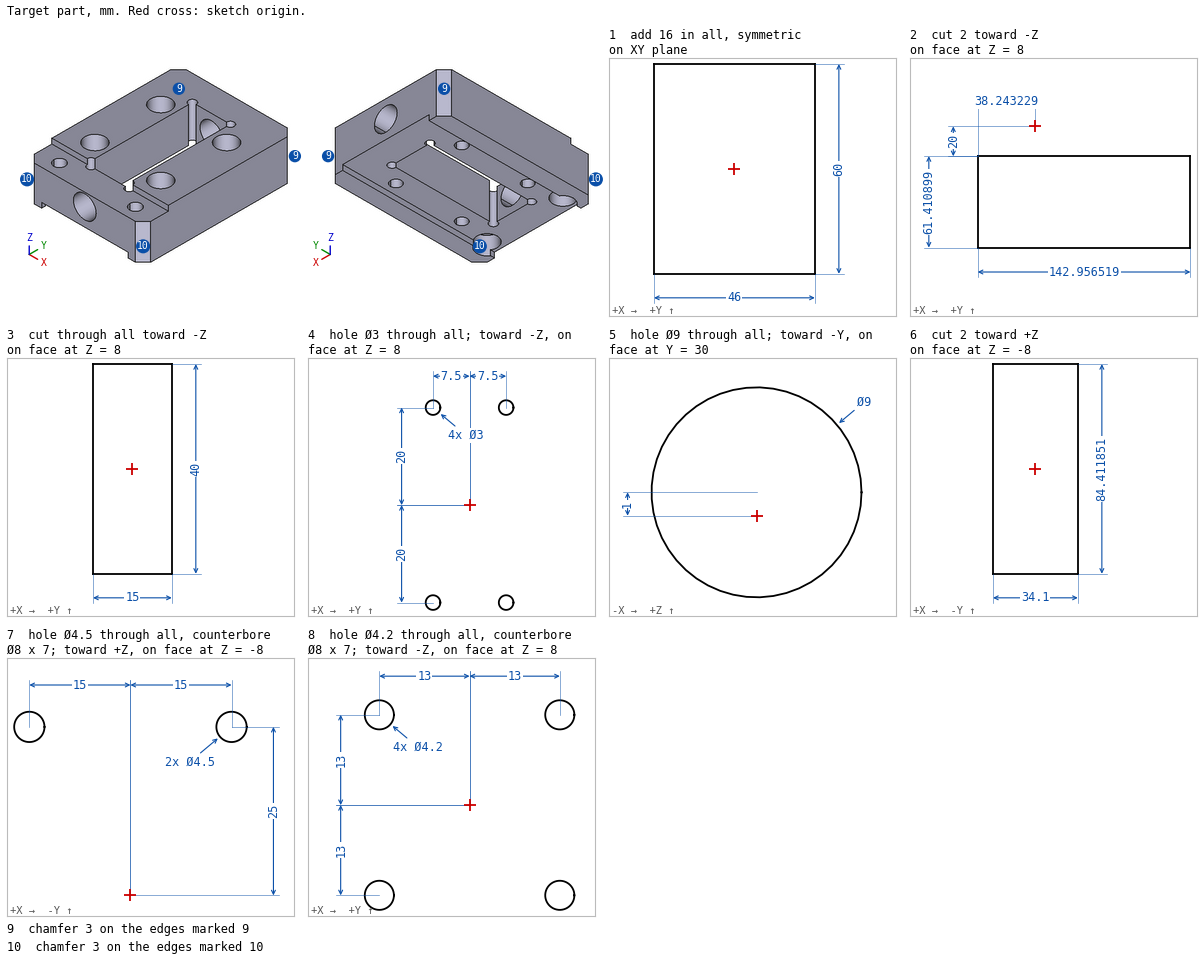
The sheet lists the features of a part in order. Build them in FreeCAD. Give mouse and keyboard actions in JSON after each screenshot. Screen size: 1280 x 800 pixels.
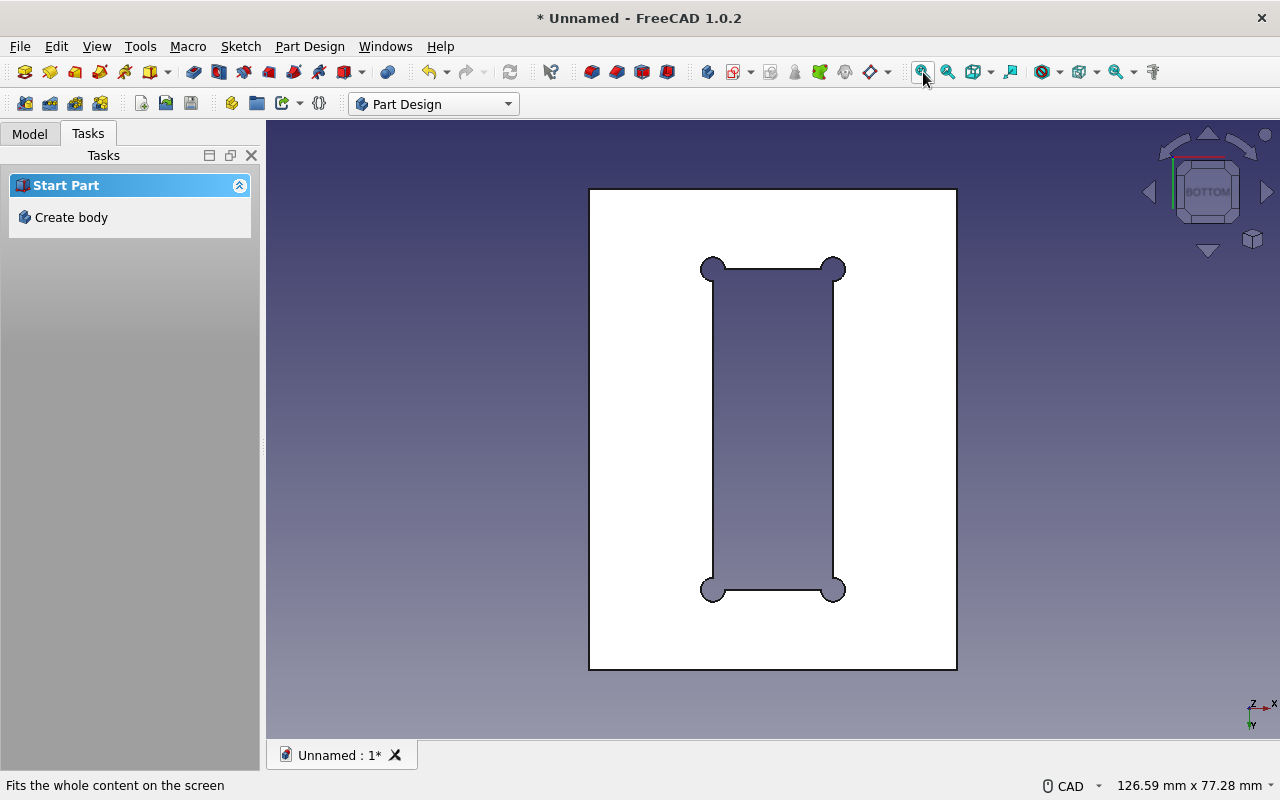
{"action": "left_click", "coordinate": [878, 497]}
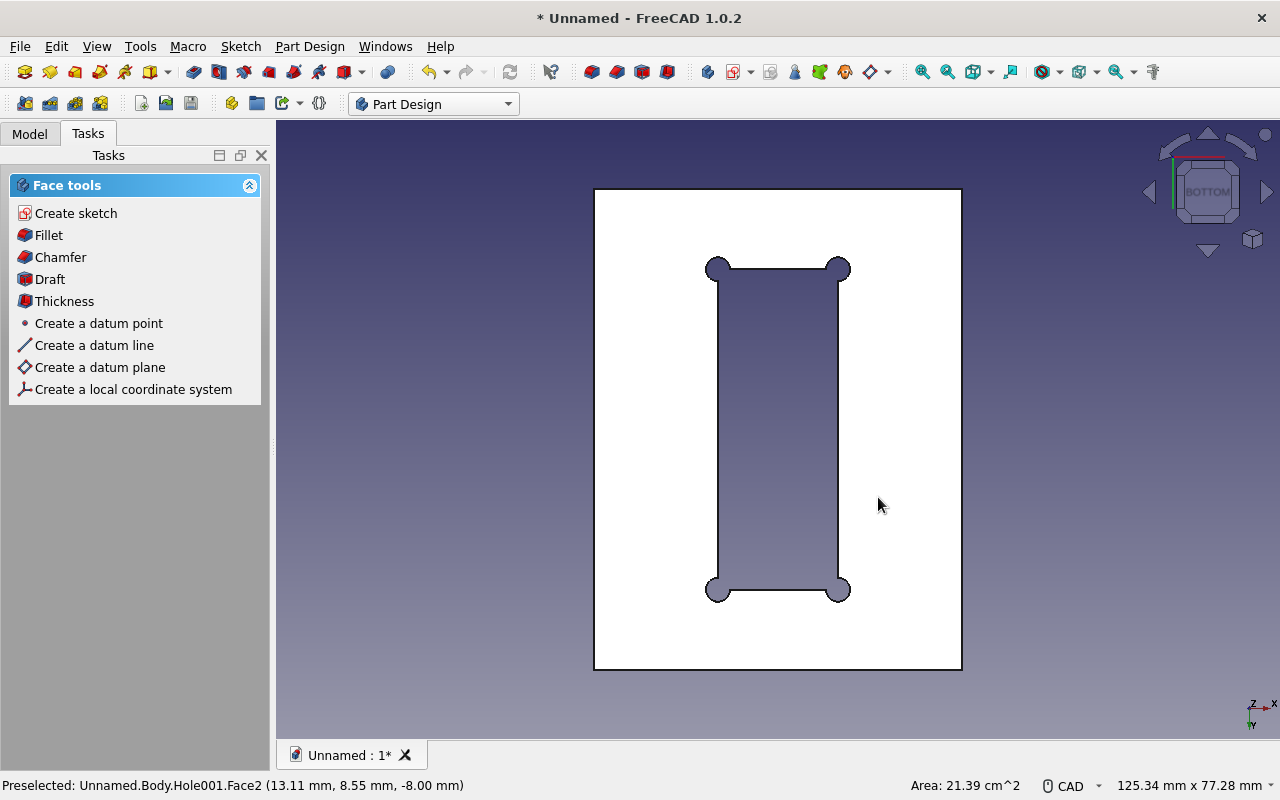
{"action": "left_click", "coordinate": [732, 72]}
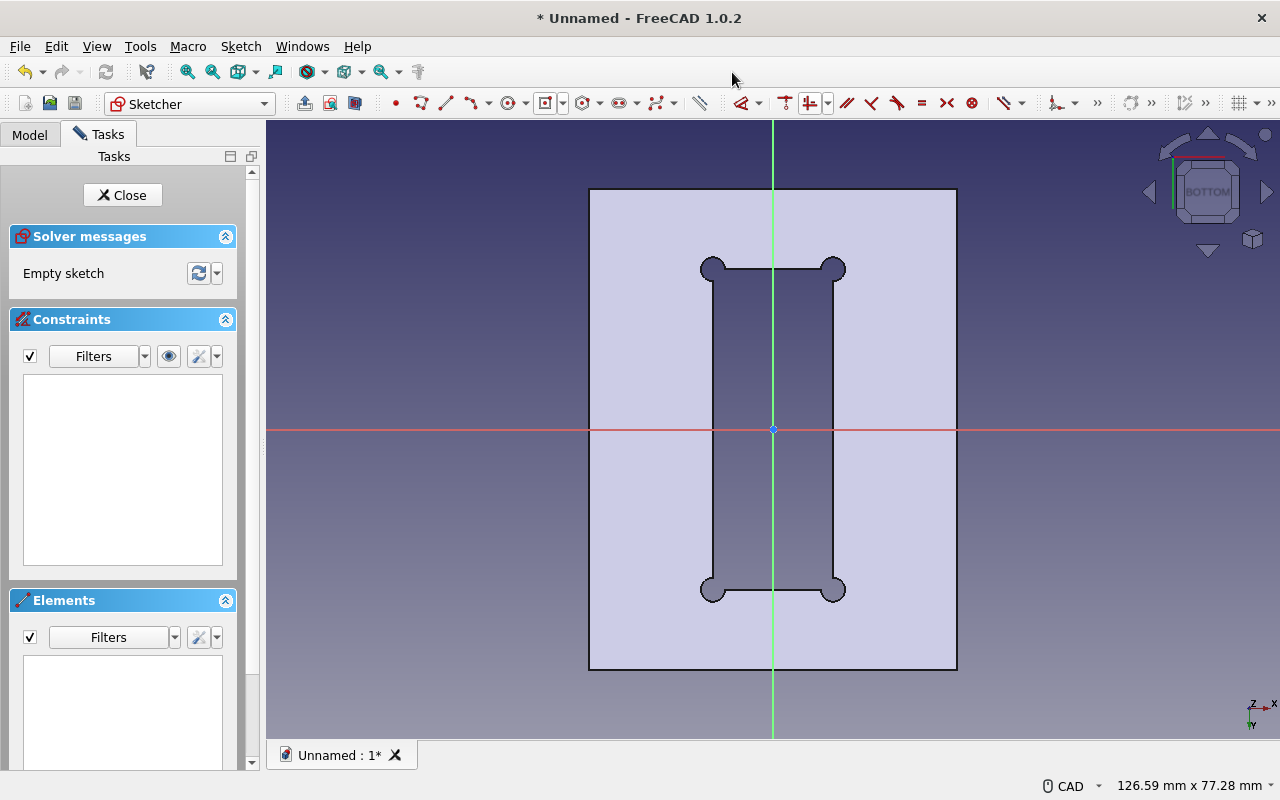
{"action": "scroll", "coordinate": [621, 430], "scroll_direction": "down", "scroll_amount": 3}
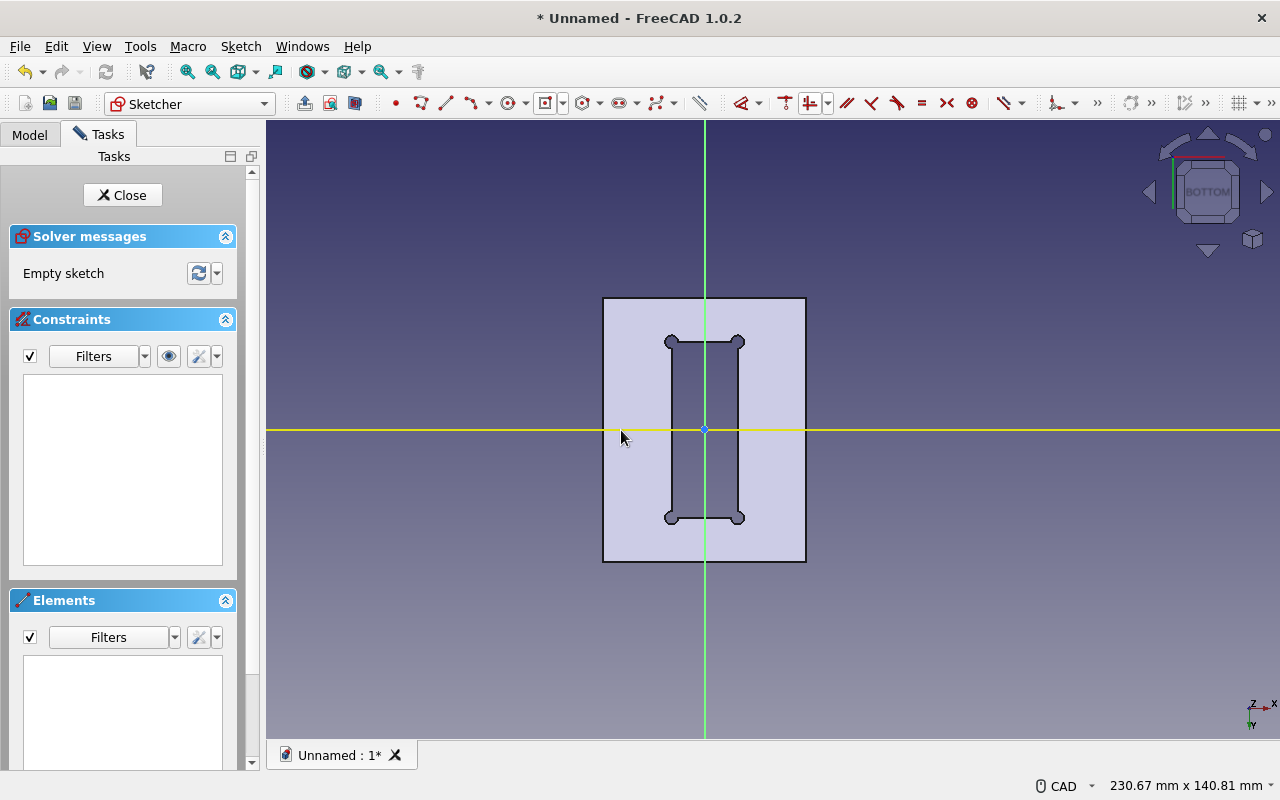
{"action": "left_click", "coordinate": [544, 104]}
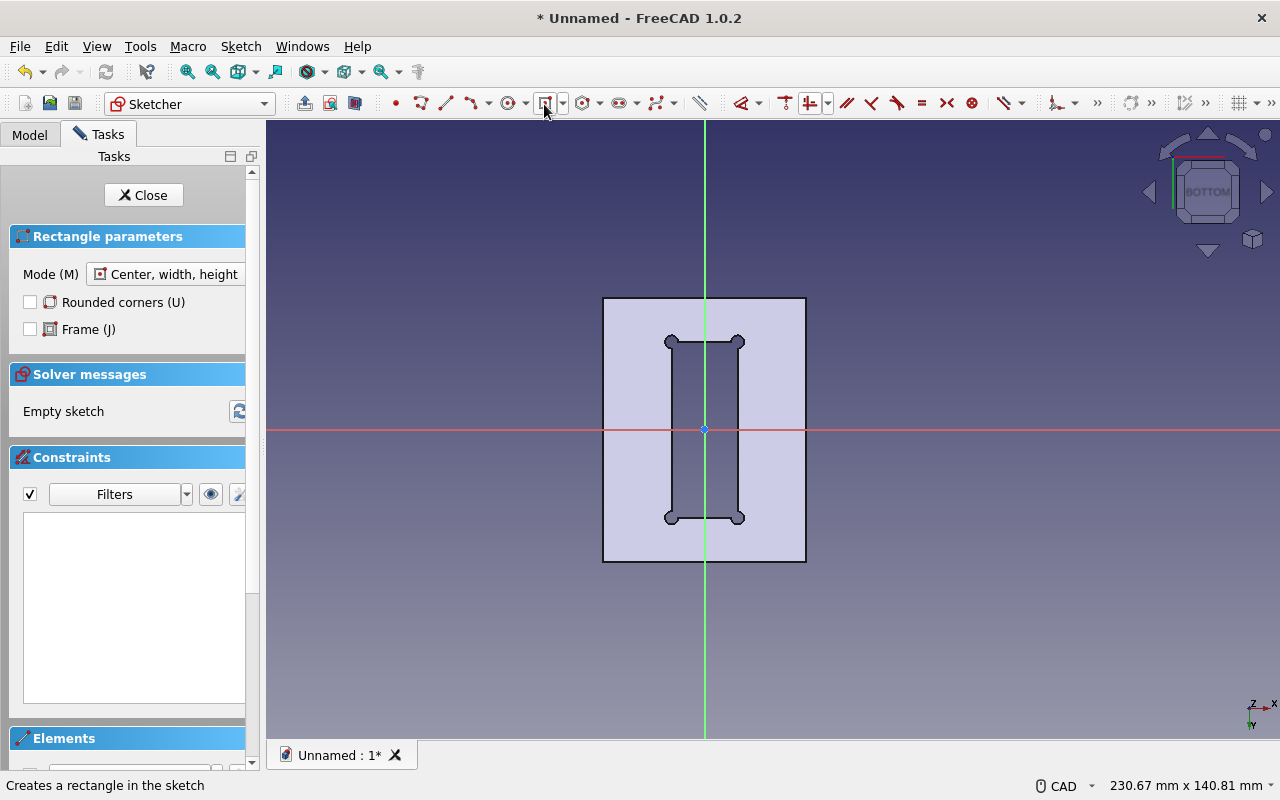
{"action": "left_click", "coordinate": [705, 430]}
{"action": "left_click", "coordinate": [780, 244]}
{"action": "key", "text": "Escape"}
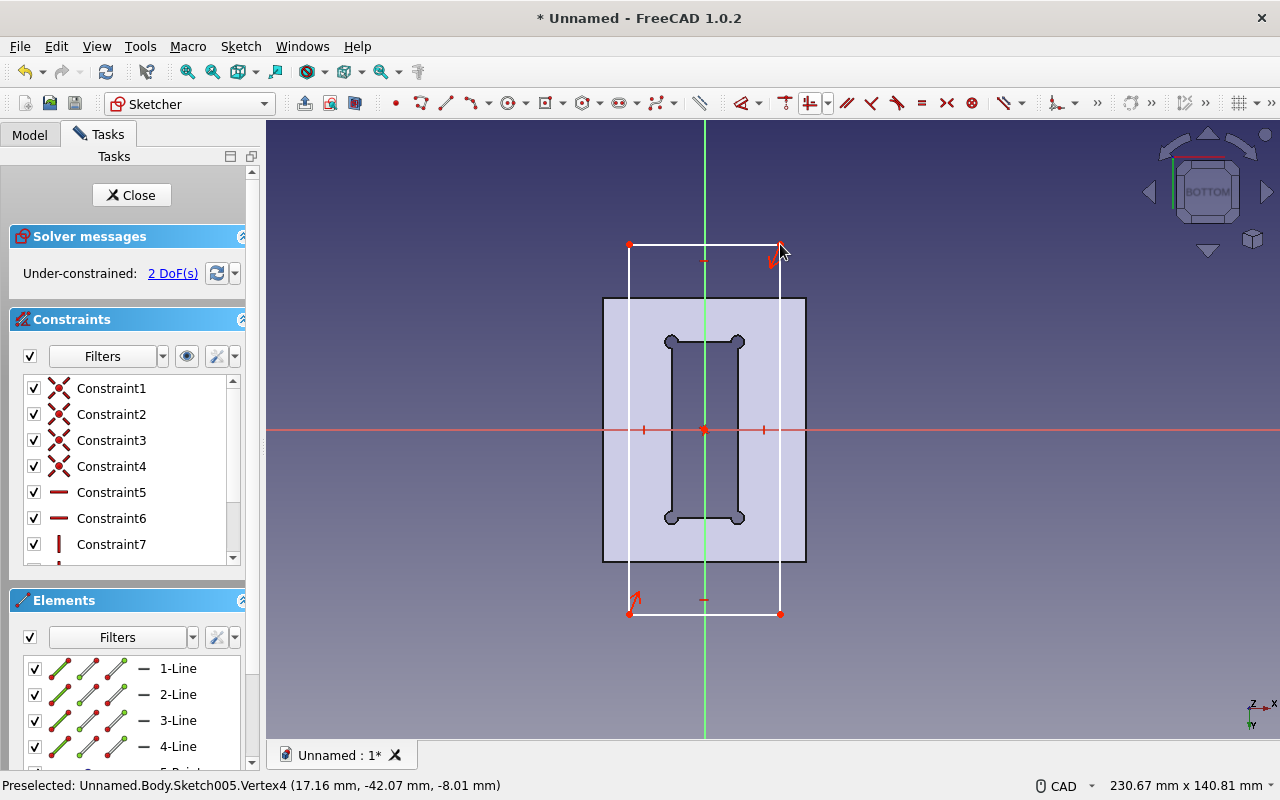
{"action": "left_click", "coordinate": [740, 104]}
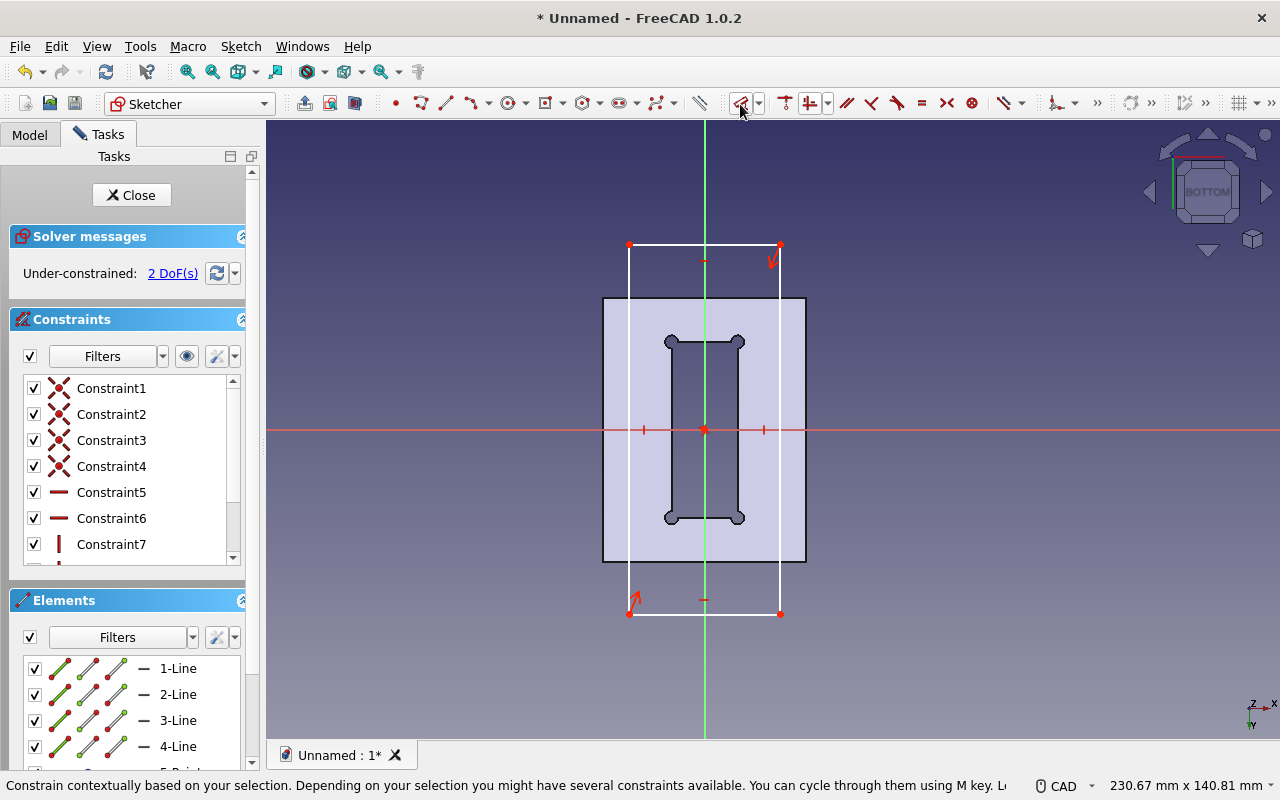
{"action": "left_click", "coordinate": [674, 615]}
{"action": "left_click", "coordinate": [670, 649]}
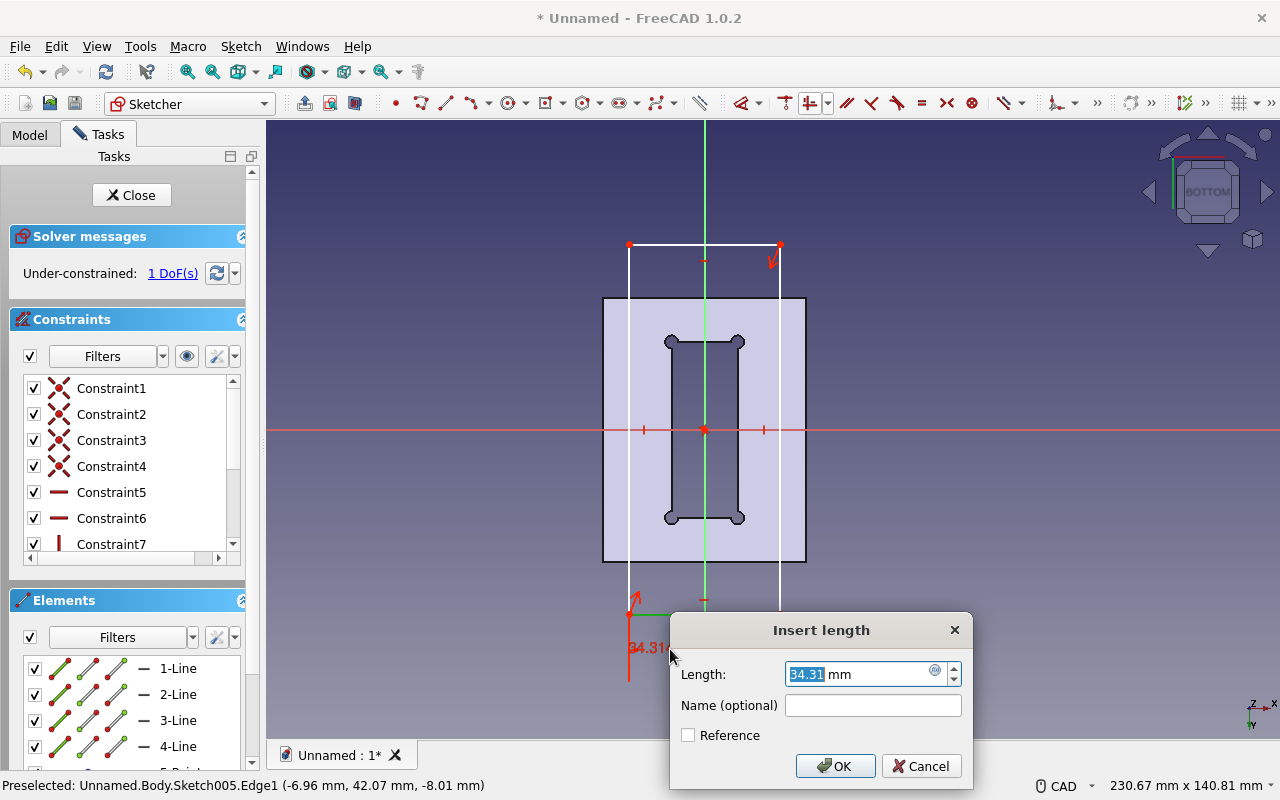
{"action": "type", "text": "34.1"}
{"action": "key", "text": "Return"}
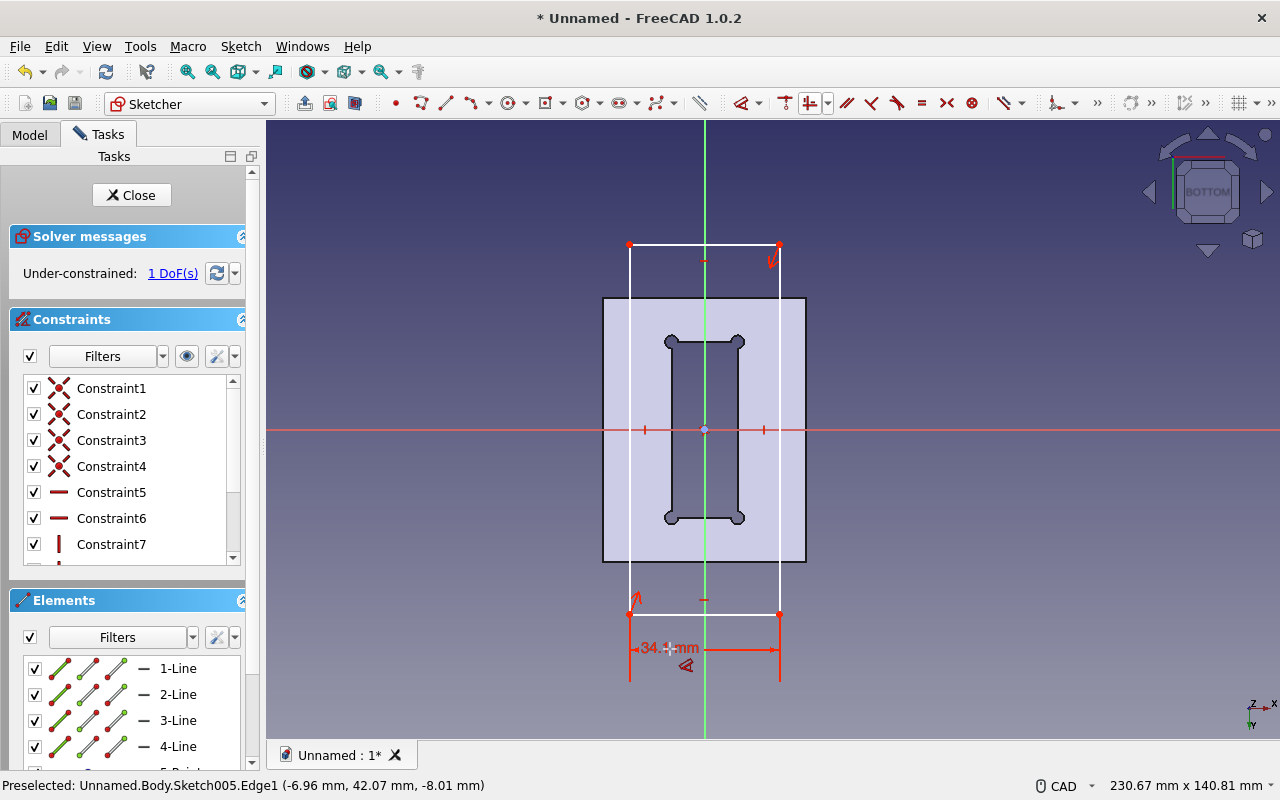
{"action": "left_click", "coordinate": [780, 504]}
{"action": "left_click", "coordinate": [814, 345]}